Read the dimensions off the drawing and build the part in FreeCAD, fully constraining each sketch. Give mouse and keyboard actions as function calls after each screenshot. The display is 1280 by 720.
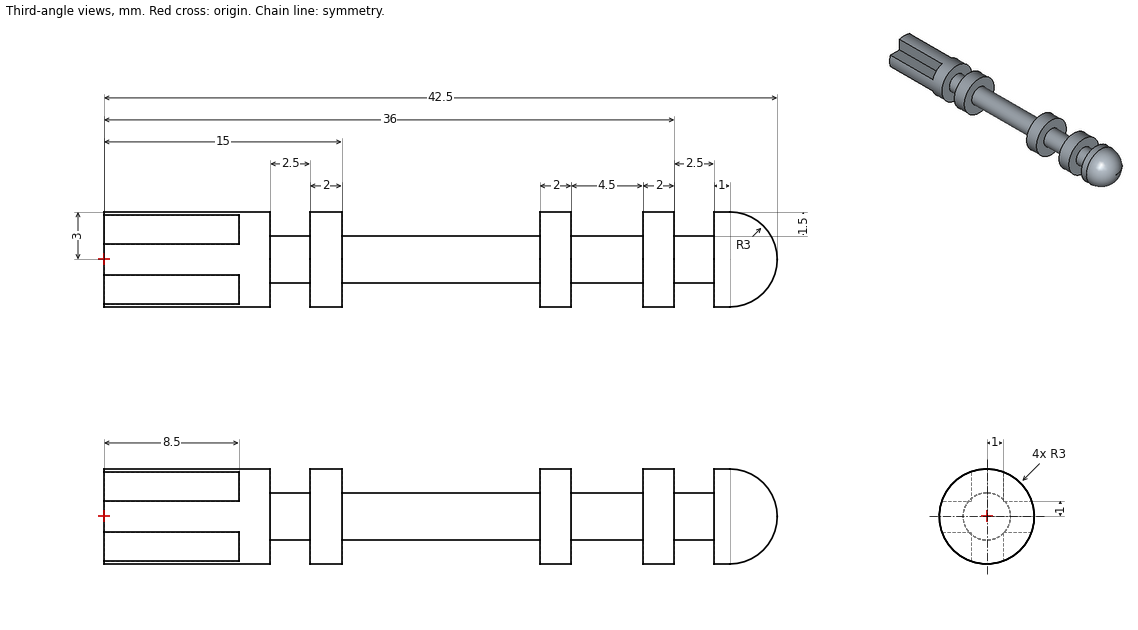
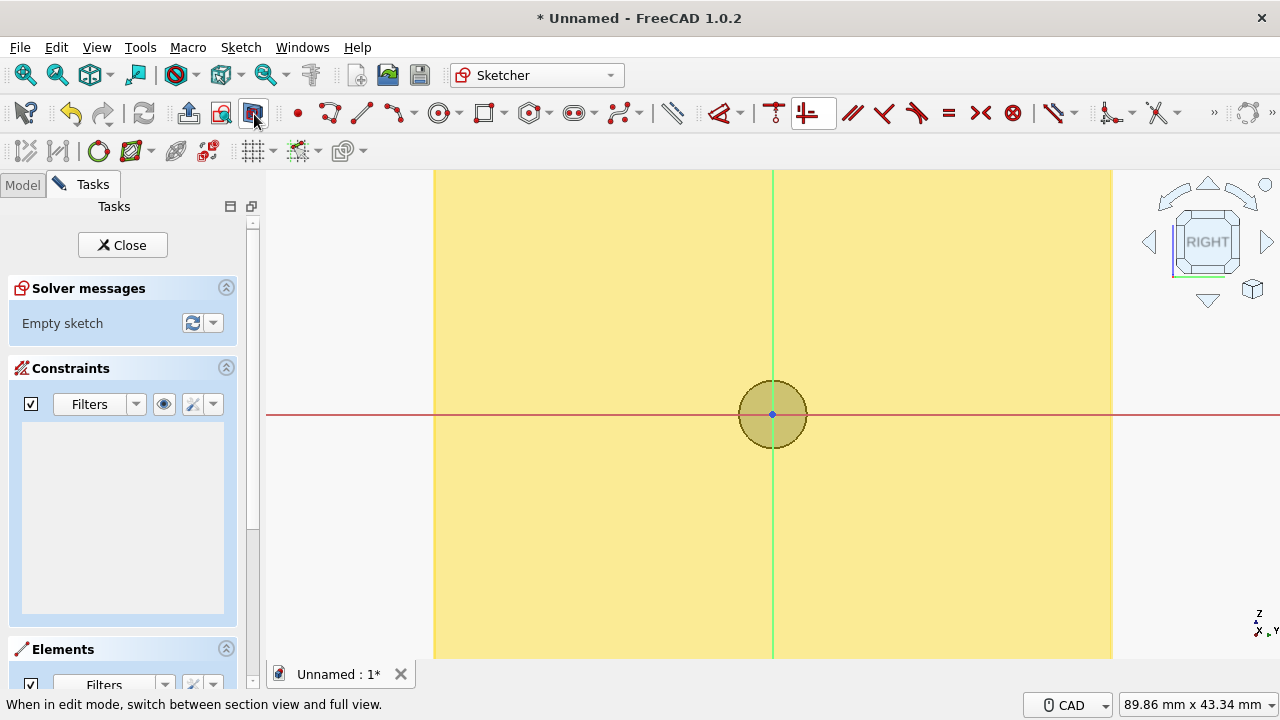
scroll(790, 414, up, 8)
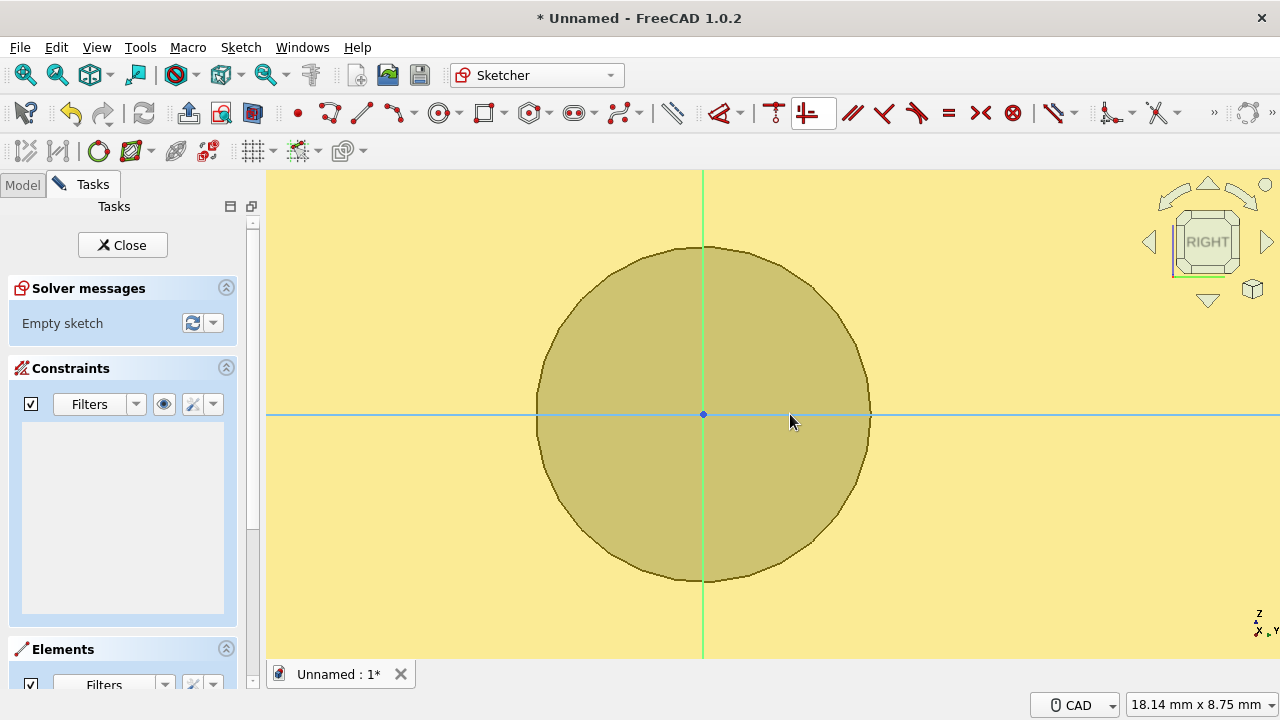
click(330, 114)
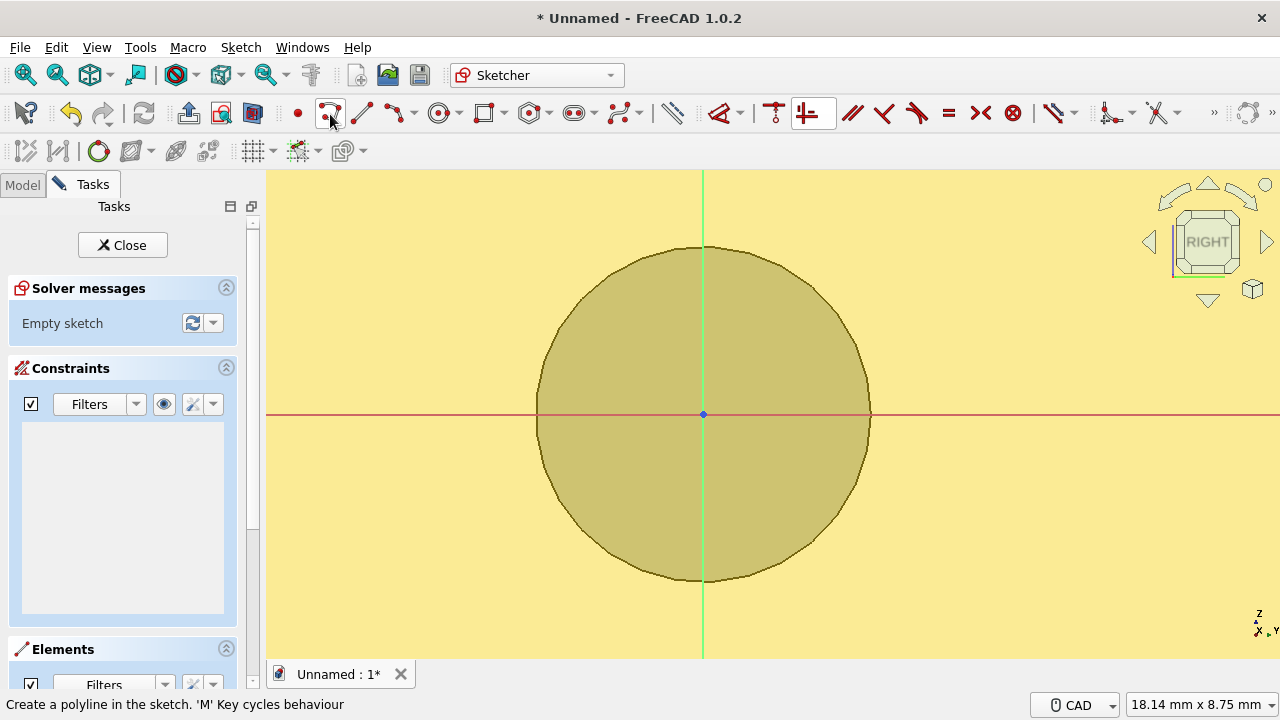
click(861, 359)
click(759, 359)
click(759, 256)
right_click(759, 256)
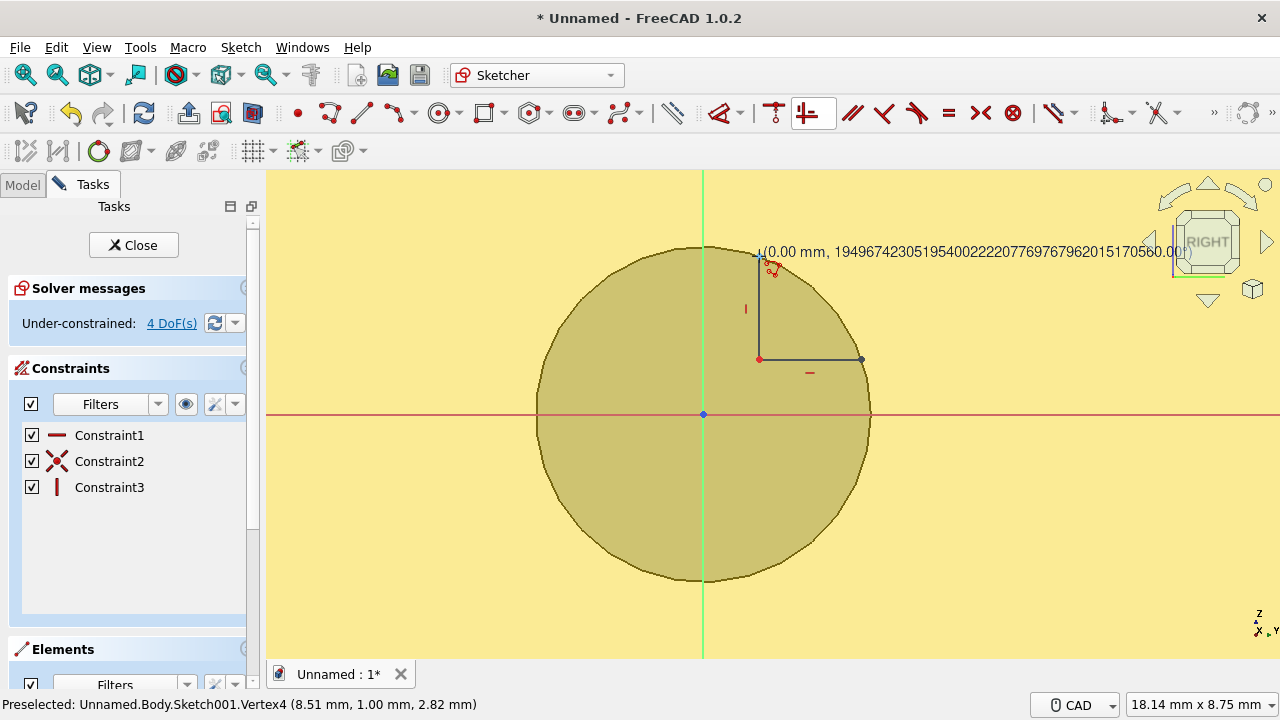
click(394, 114)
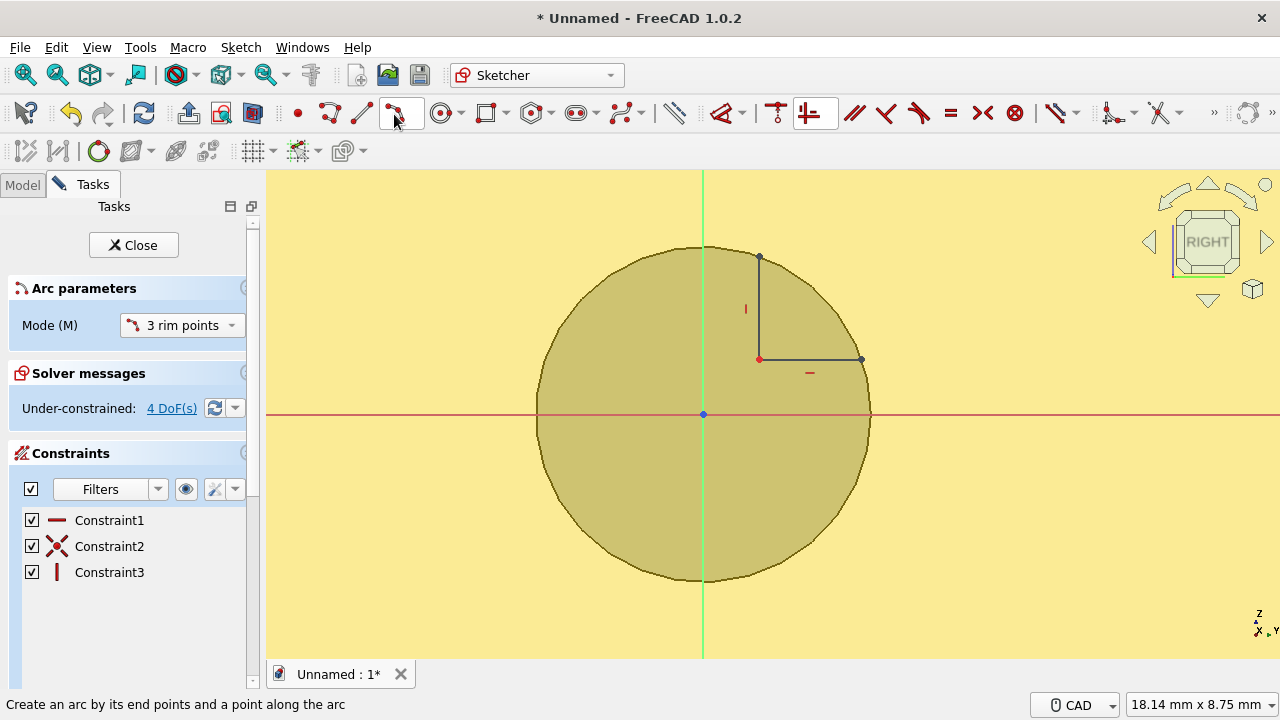
click(759, 257)
click(861, 360)
click(822, 296)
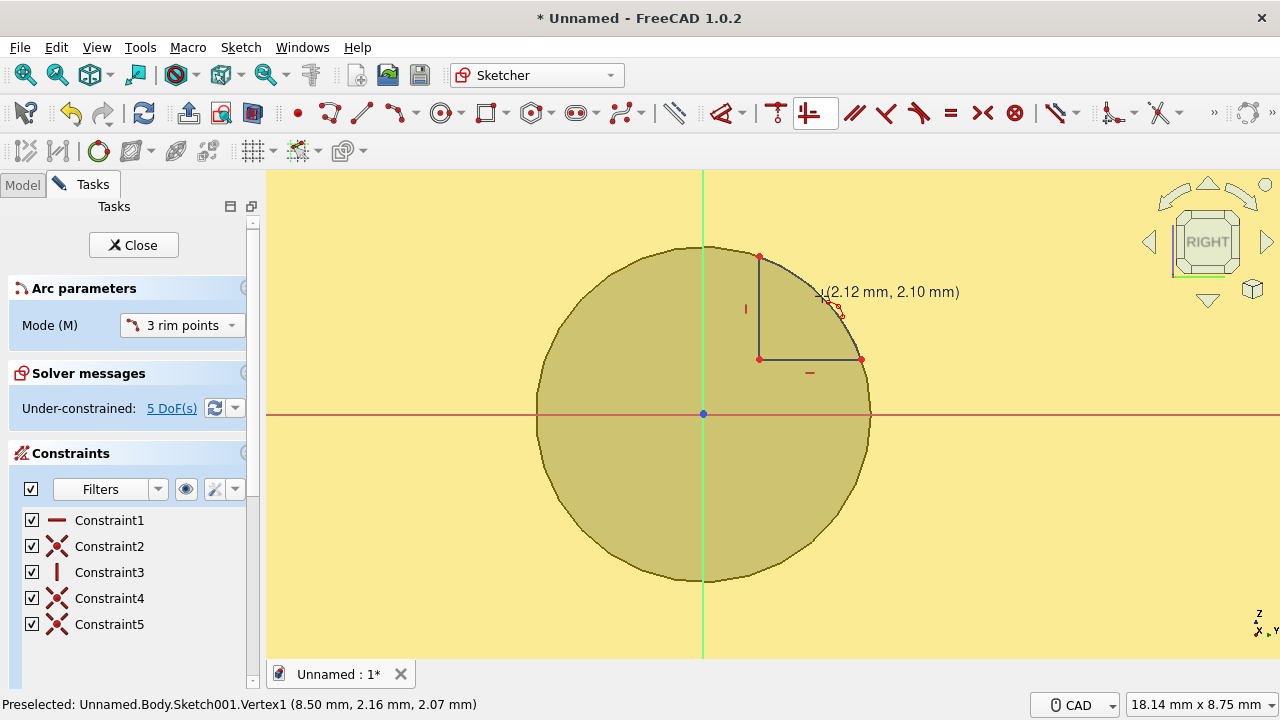
click(330, 114)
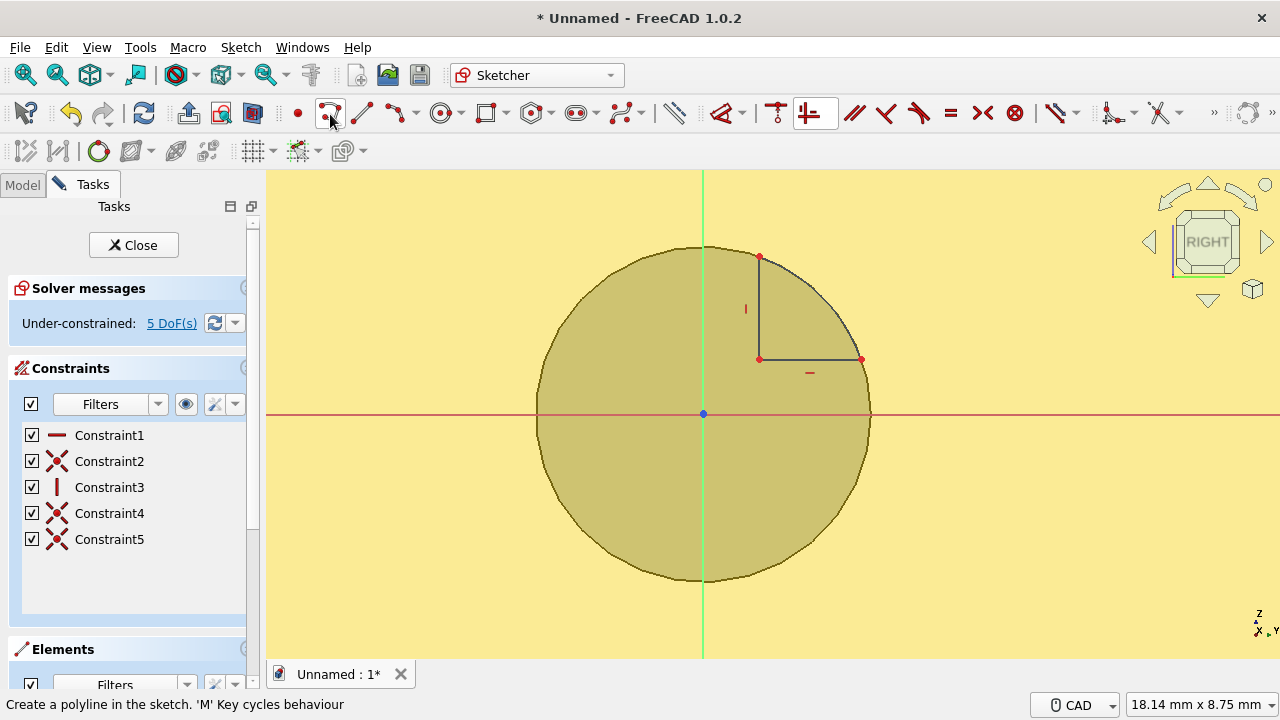
click(647, 256)
click(647, 359)
click(545, 359)
right_click(545, 359)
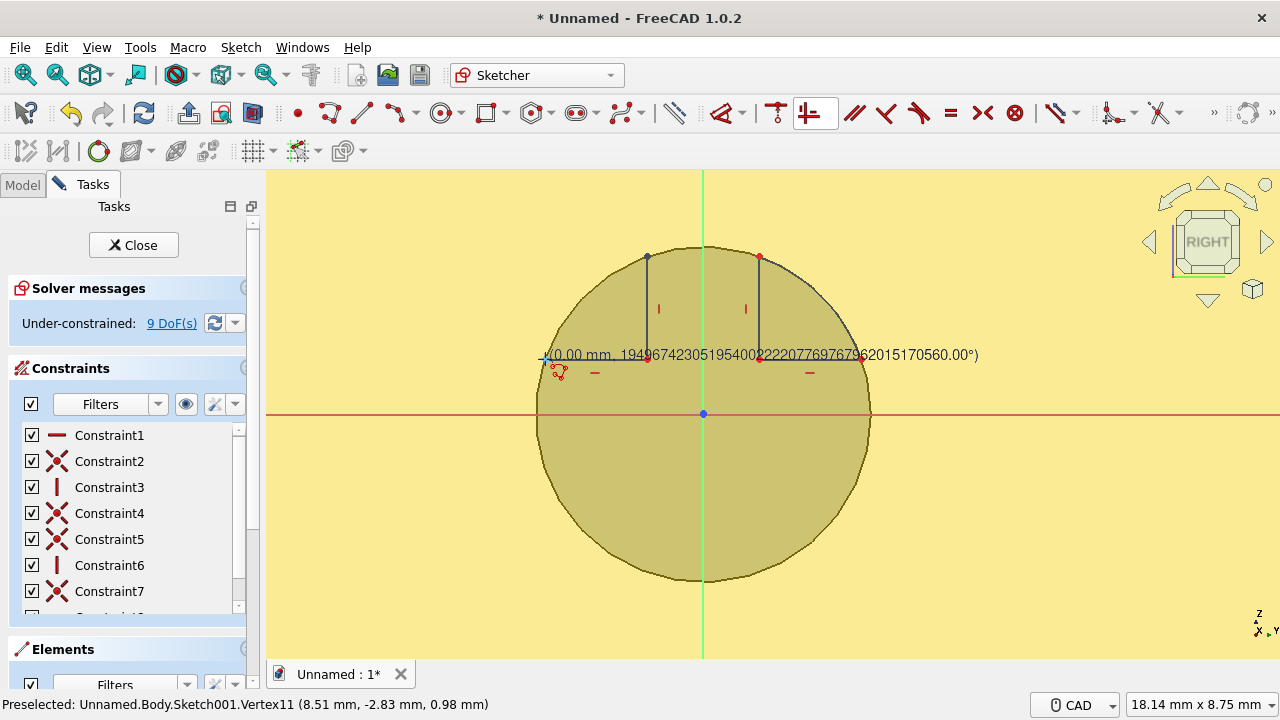
click(396, 114)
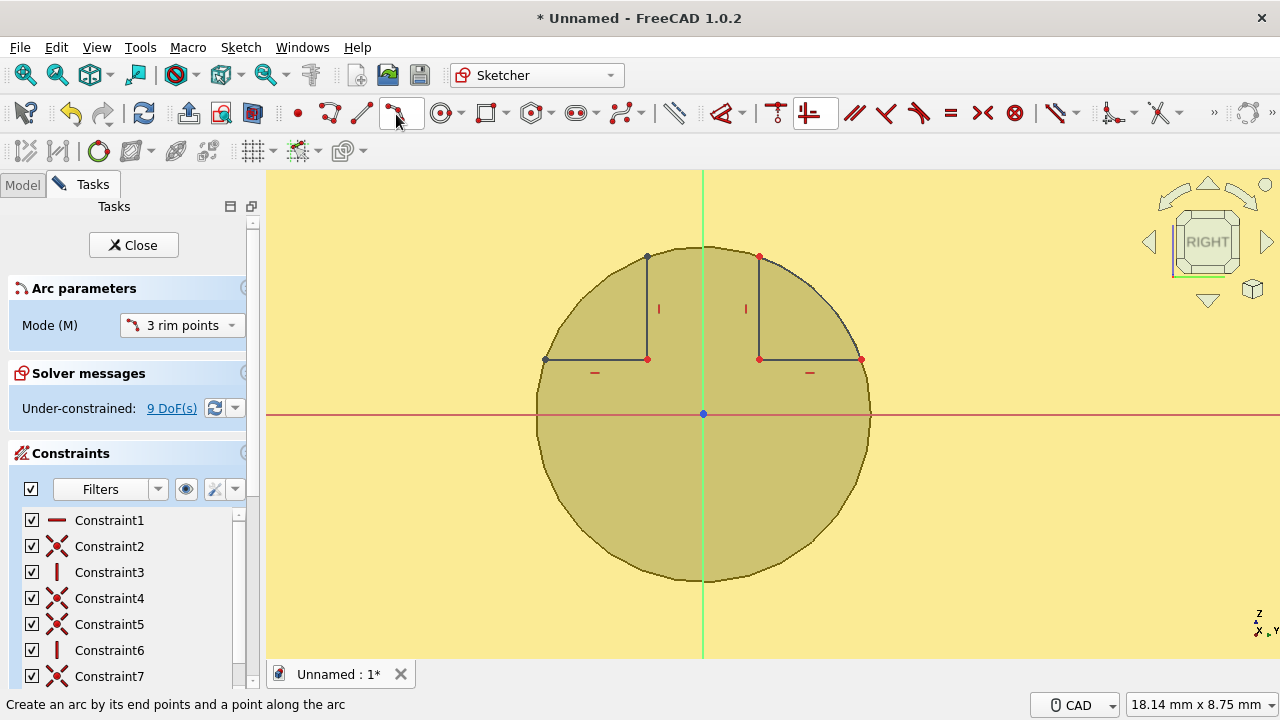
click(545, 360)
click(647, 257)
click(585, 296)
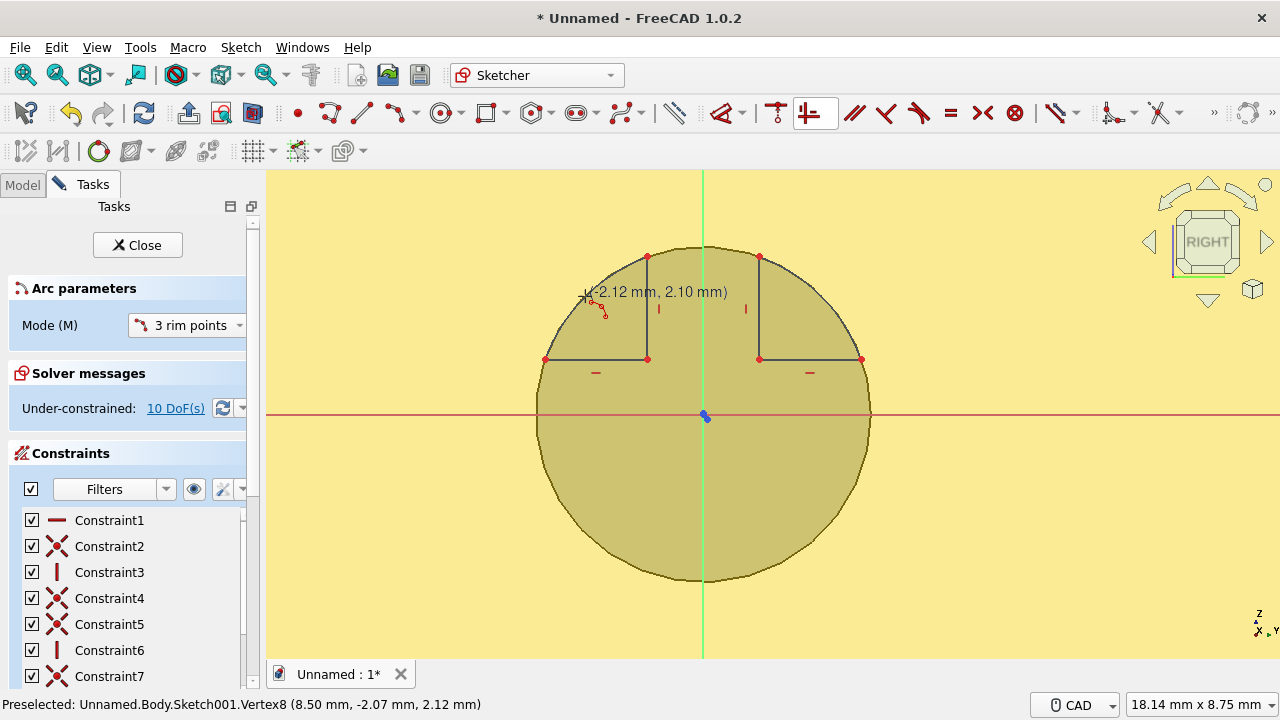
click(330, 114)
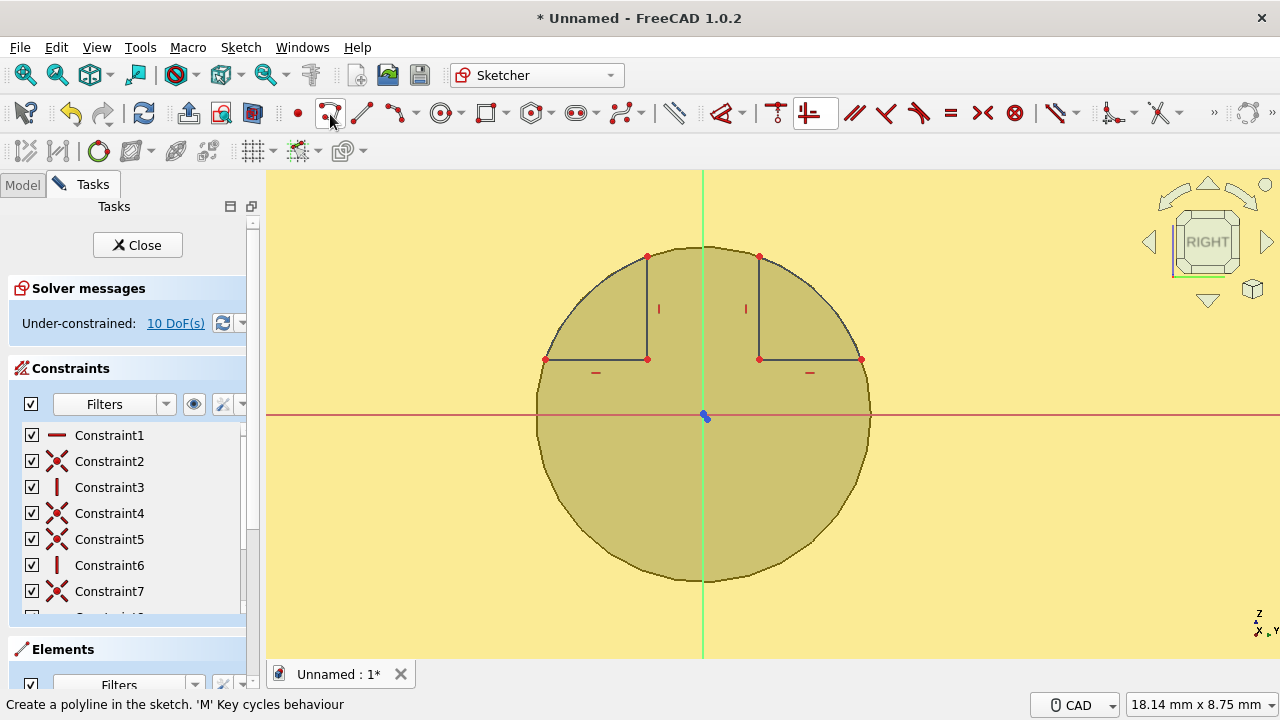
click(759, 573)
click(759, 470)
click(861, 470)
right_click(861, 470)